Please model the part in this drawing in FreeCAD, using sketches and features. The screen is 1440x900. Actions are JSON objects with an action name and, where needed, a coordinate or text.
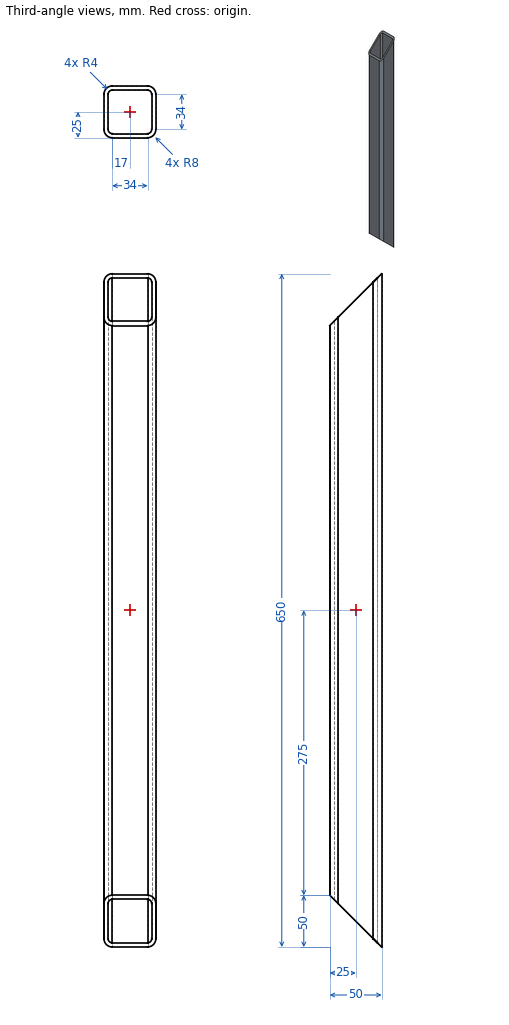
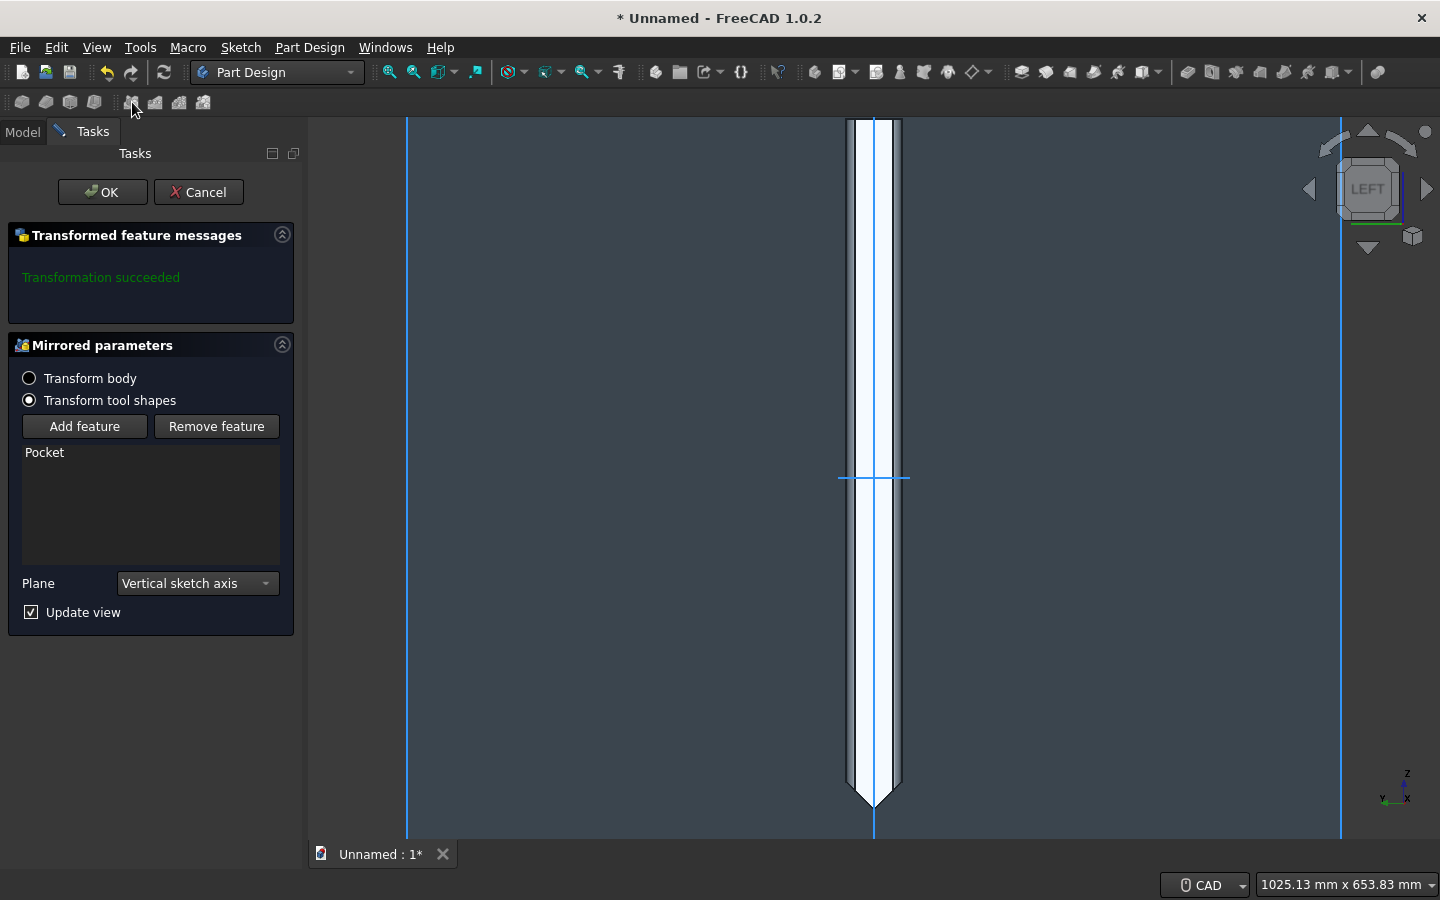
{"action": "left_click", "coordinate": [198, 584]}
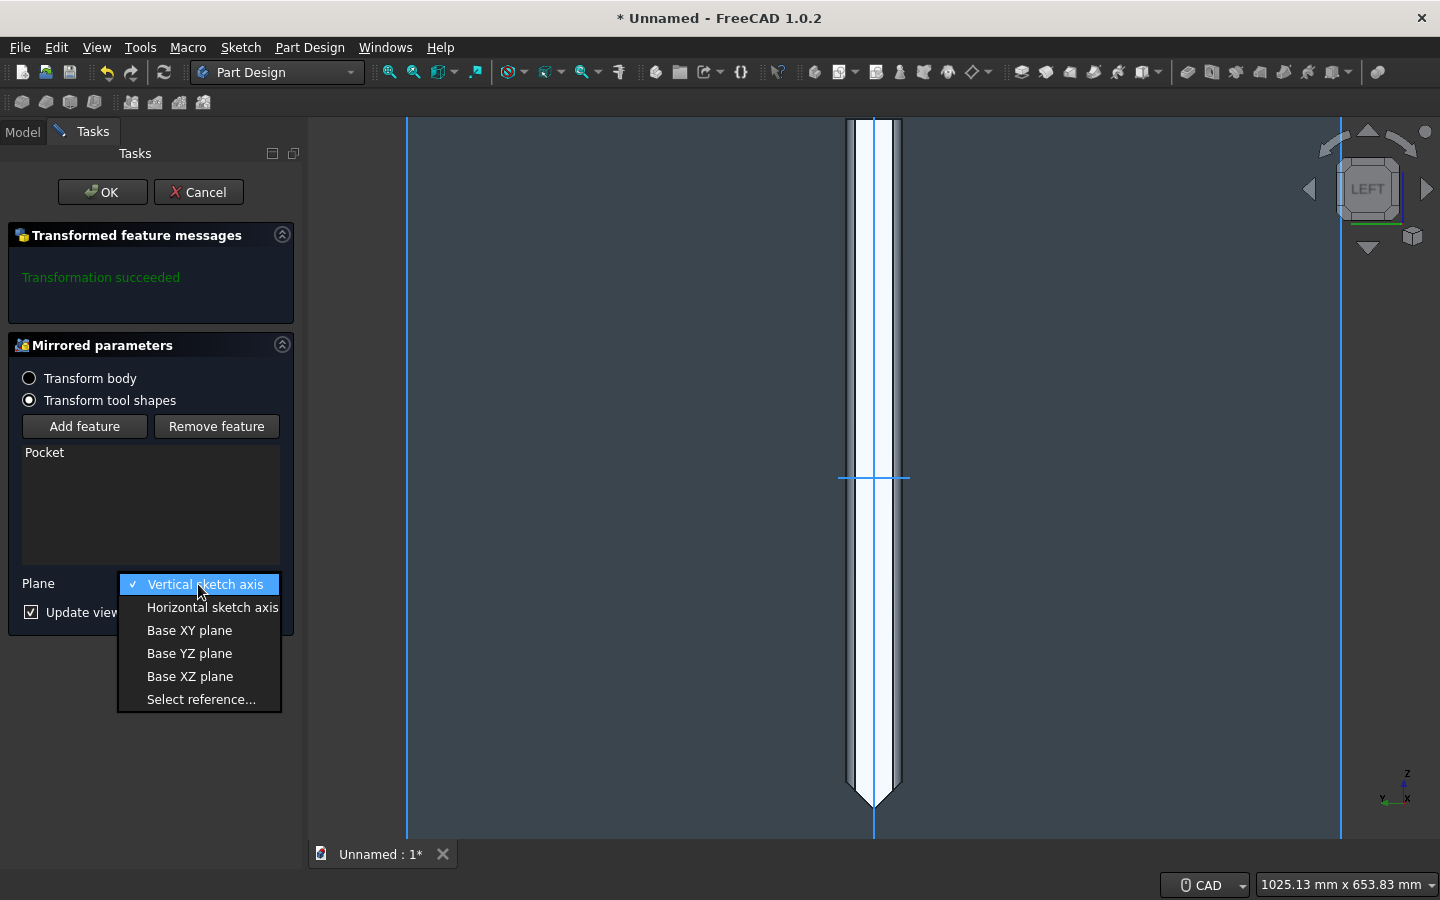
{"action": "left_click", "coordinate": [198, 630]}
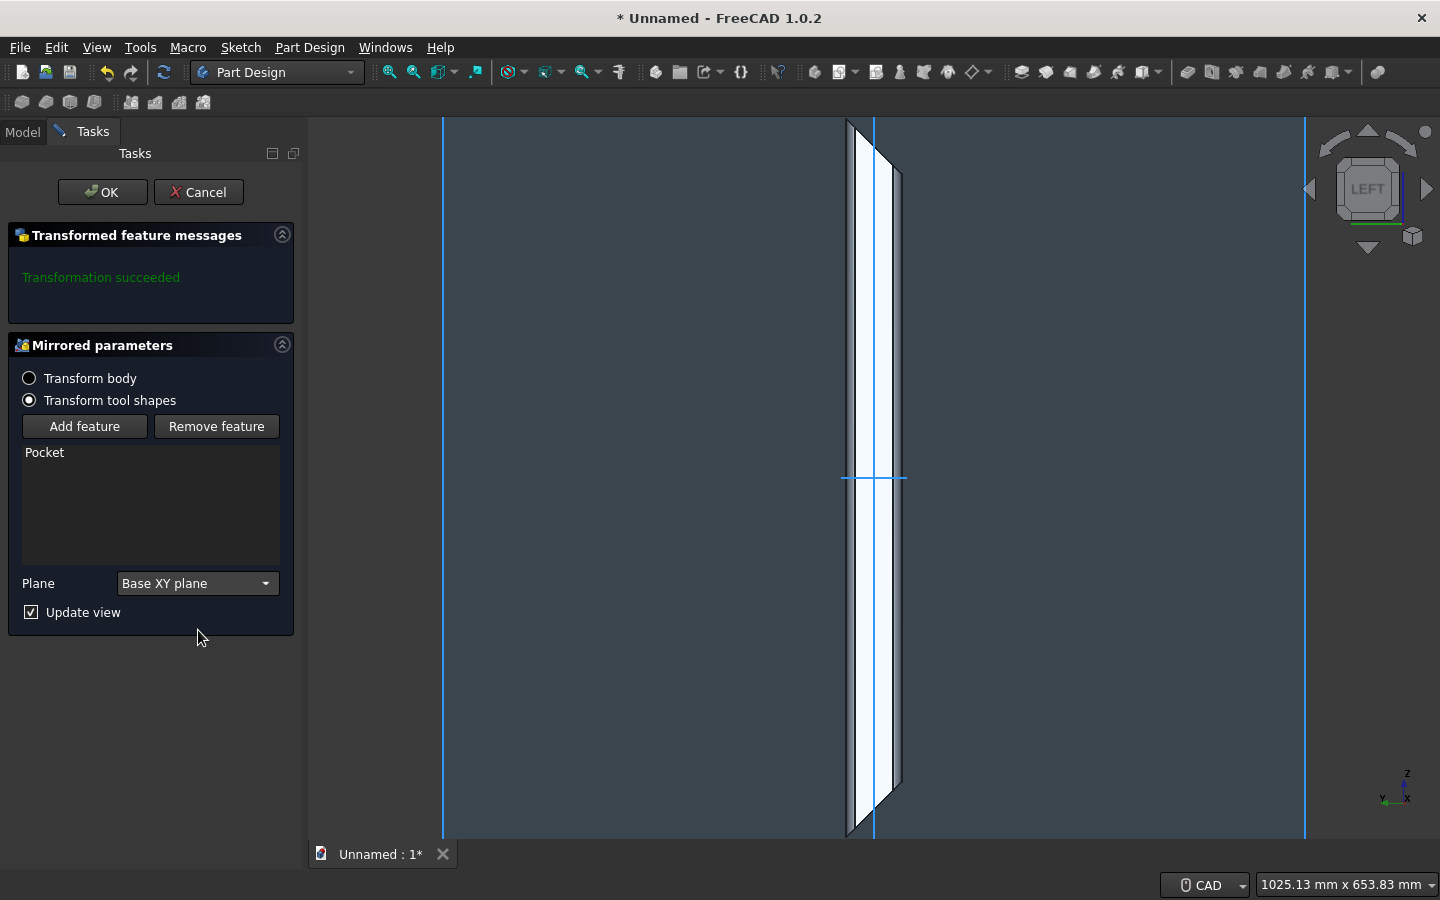
{"action": "left_click", "coordinate": [103, 192]}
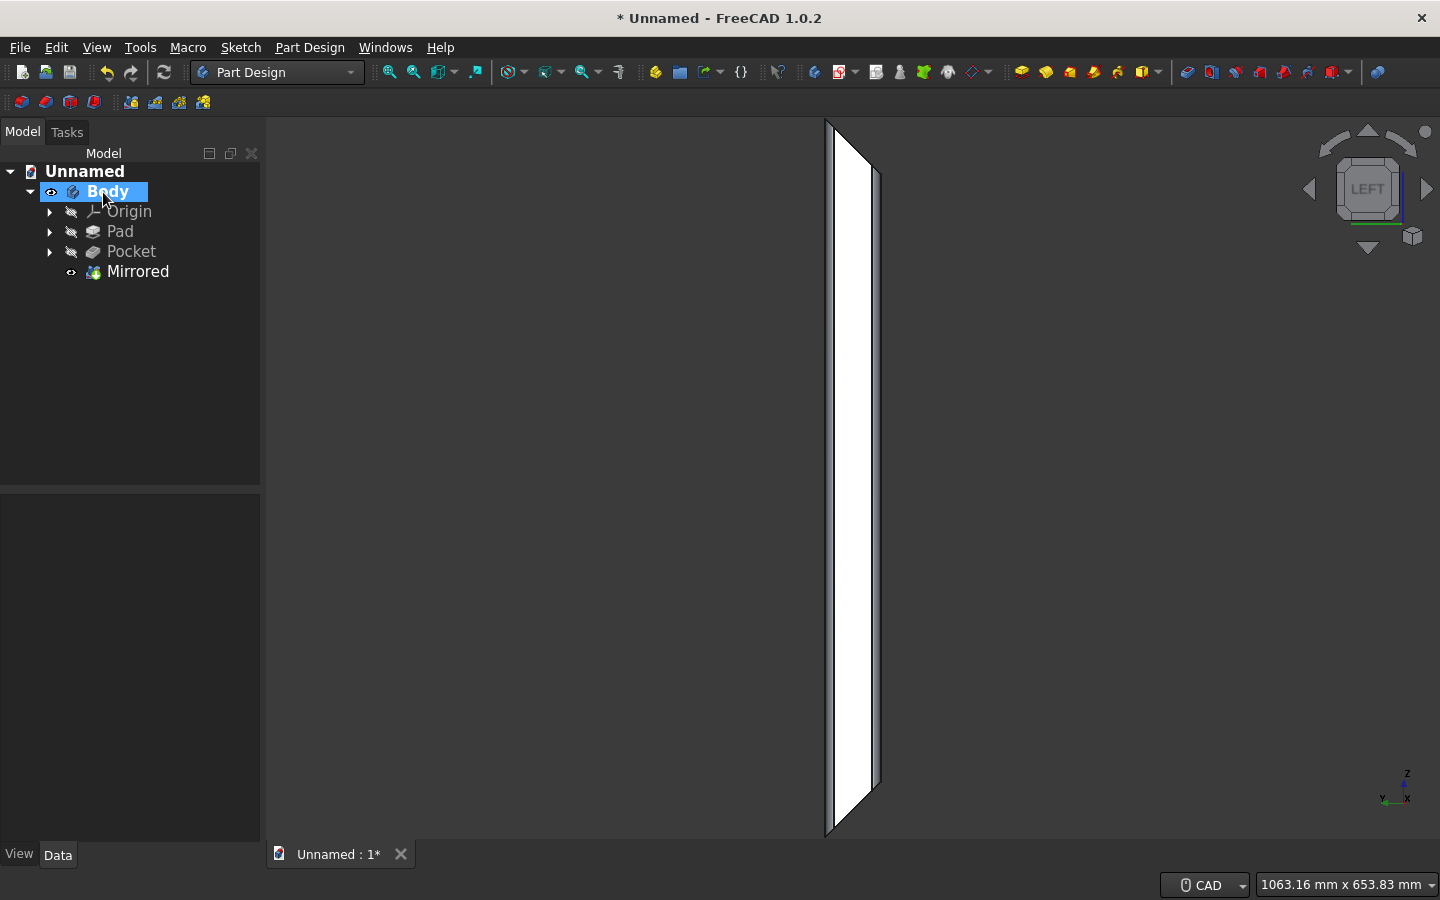
{"action": "key", "text": "0"}